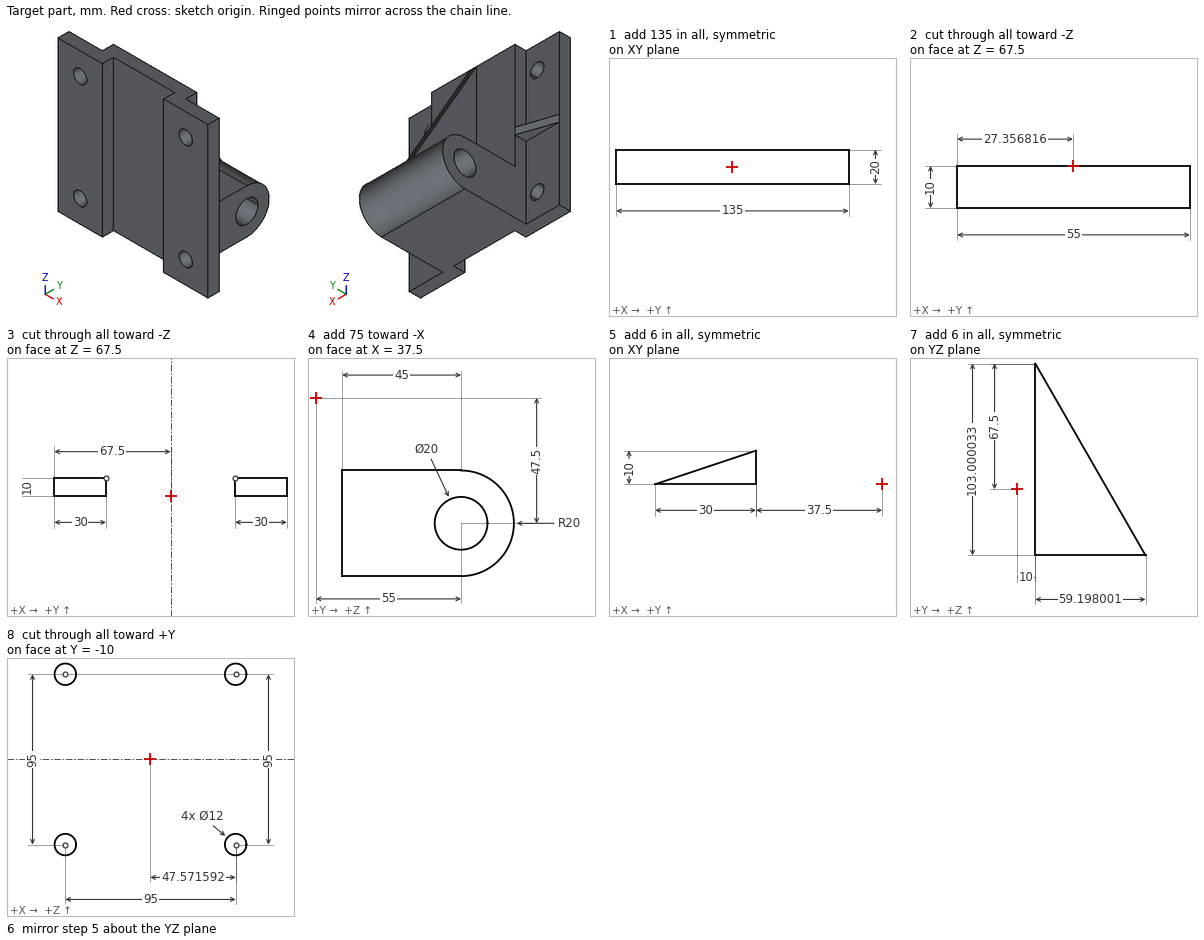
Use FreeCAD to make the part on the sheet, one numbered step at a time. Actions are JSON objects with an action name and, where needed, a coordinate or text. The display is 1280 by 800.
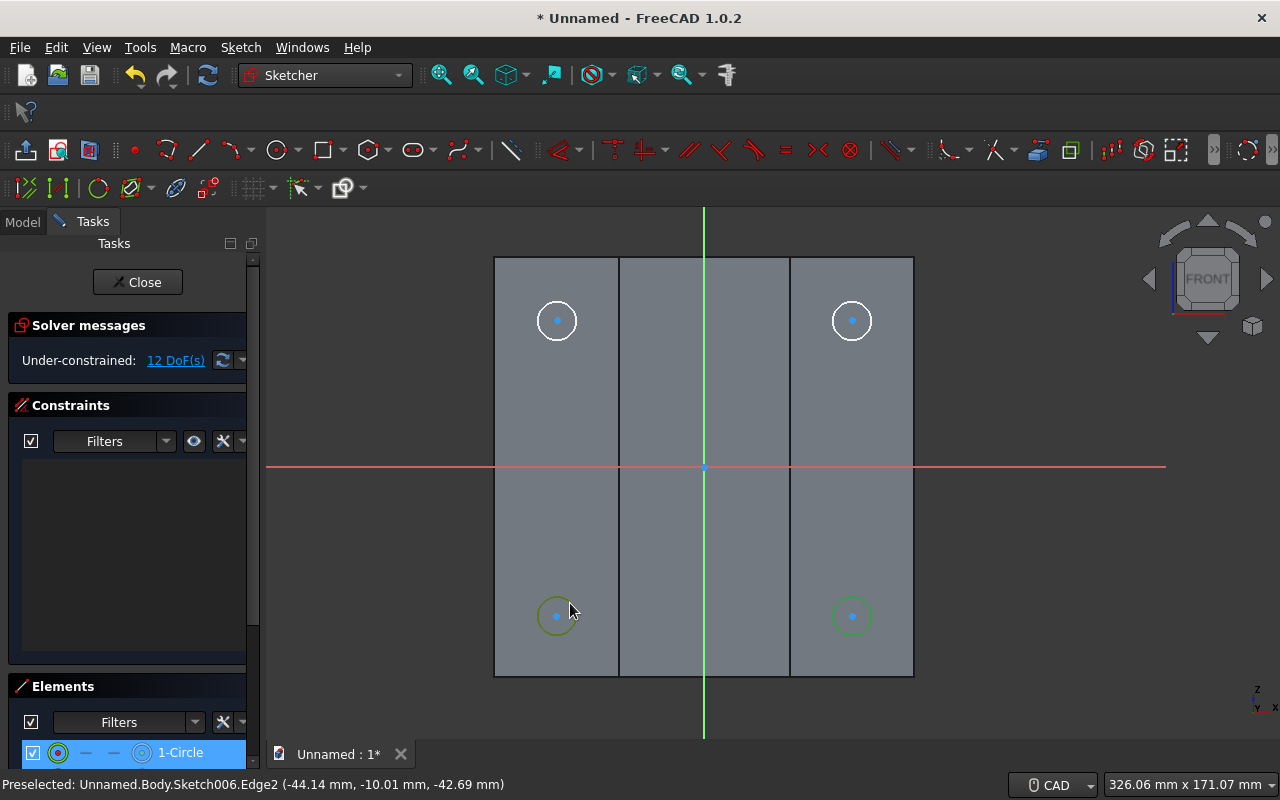
{"action": "left_click", "coordinate": [570, 307]}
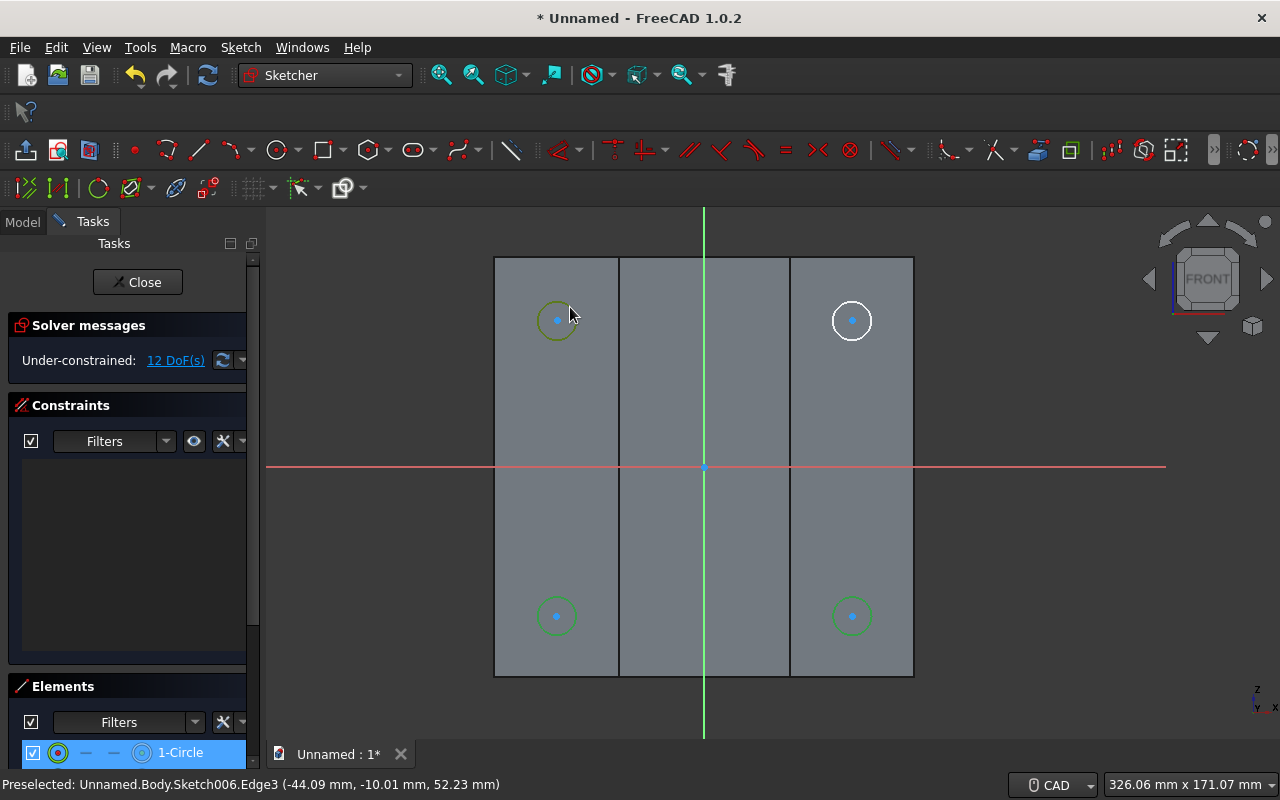
{"action": "left_click", "coordinate": [865, 307]}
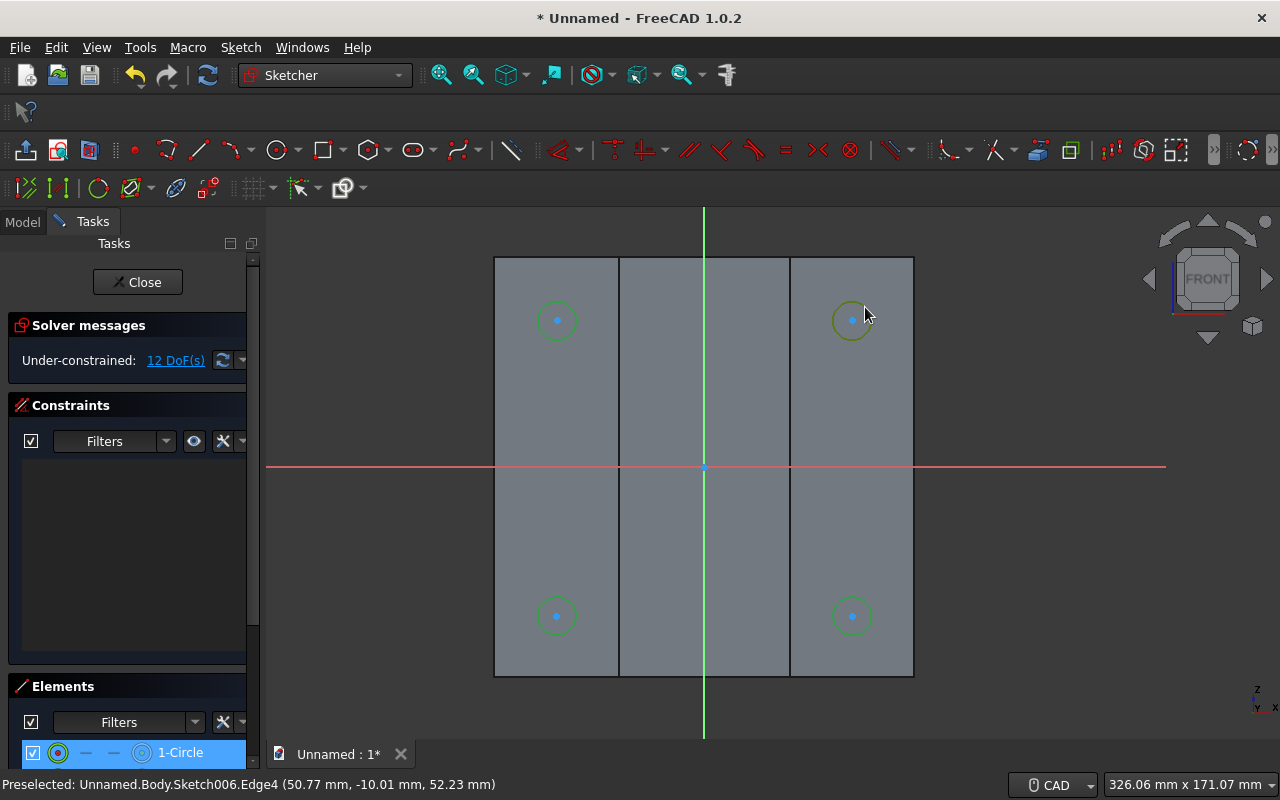
{"action": "left_click", "coordinate": [786, 150]}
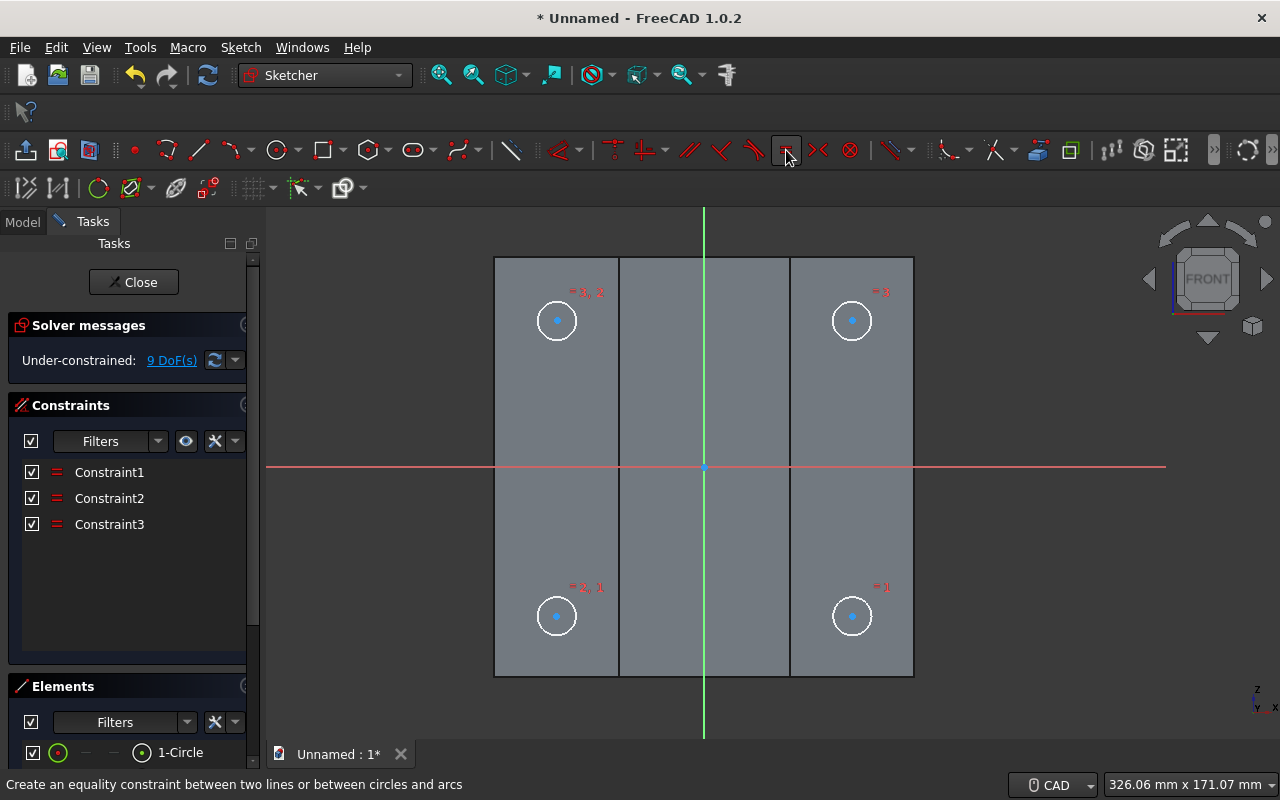
{"action": "left_click", "coordinate": [557, 616]}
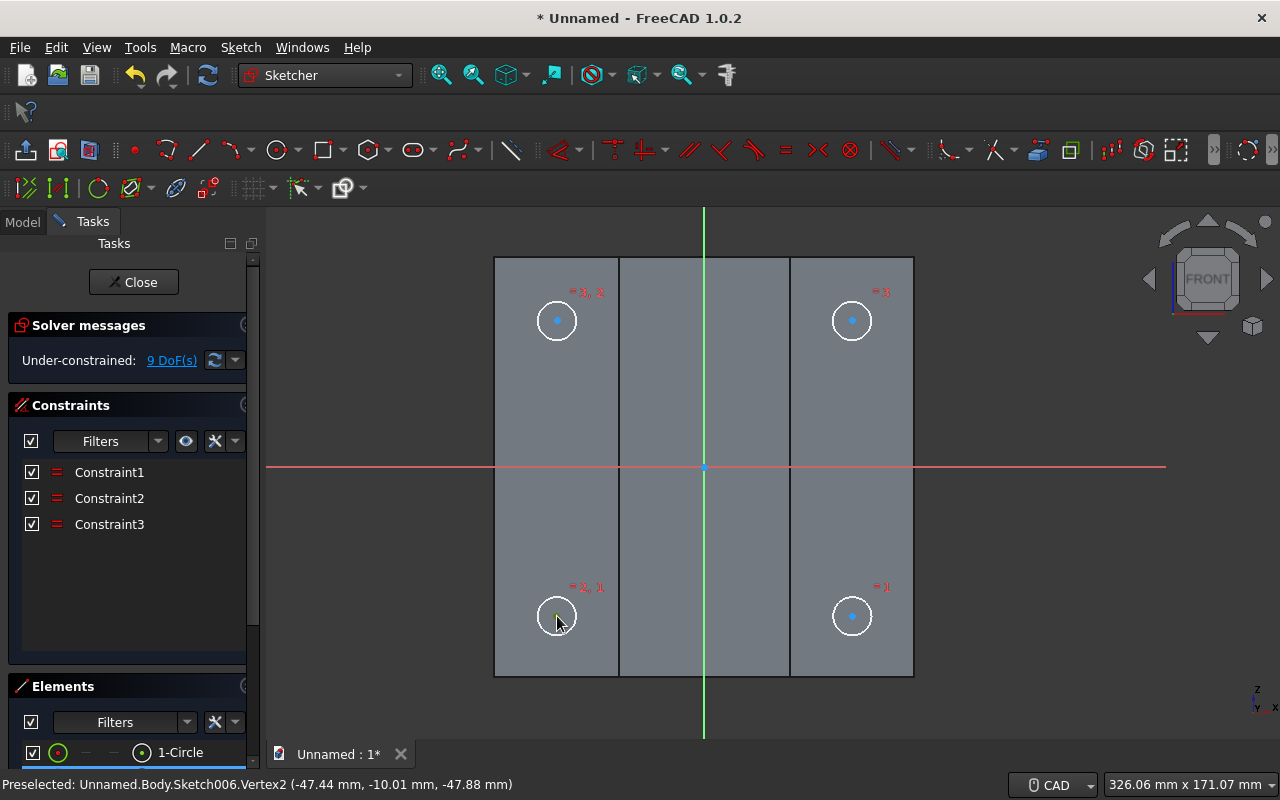
{"action": "left_click", "coordinate": [557, 321]}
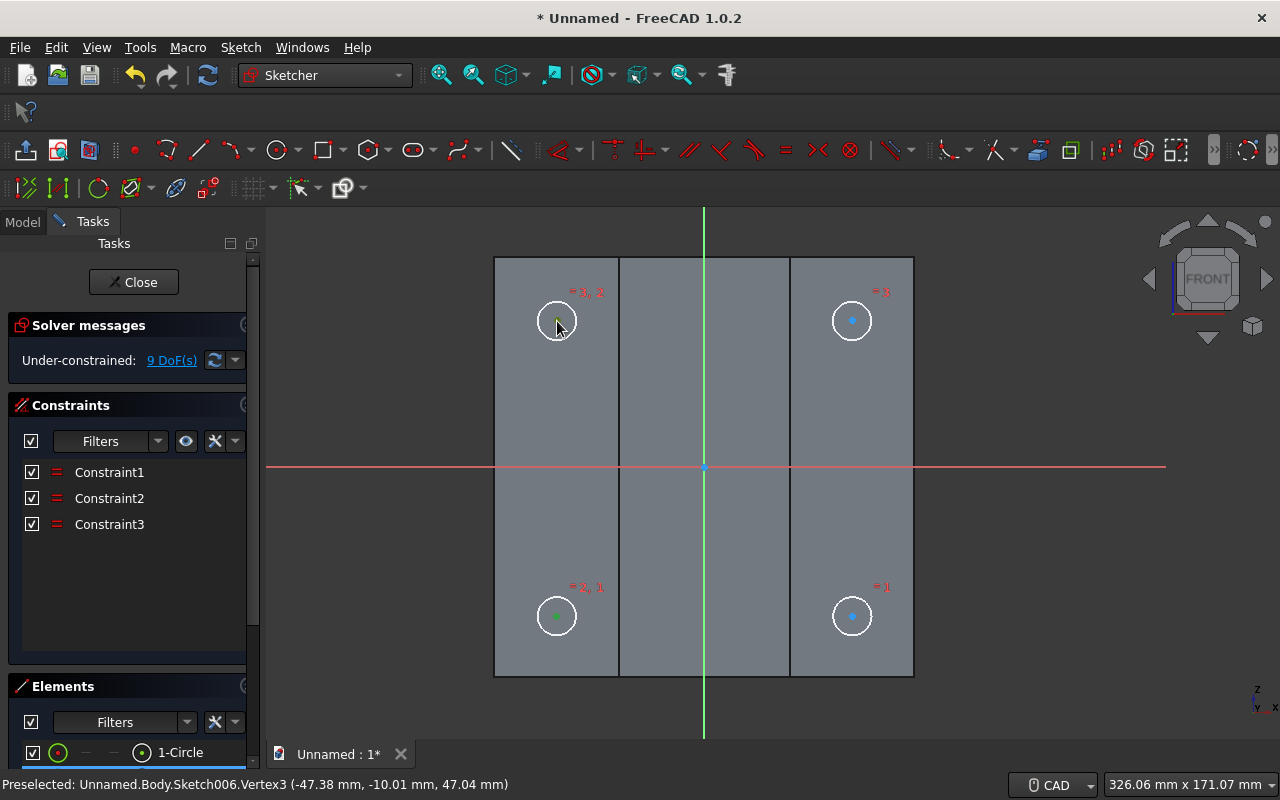
{"action": "left_click", "coordinate": [353, 467]}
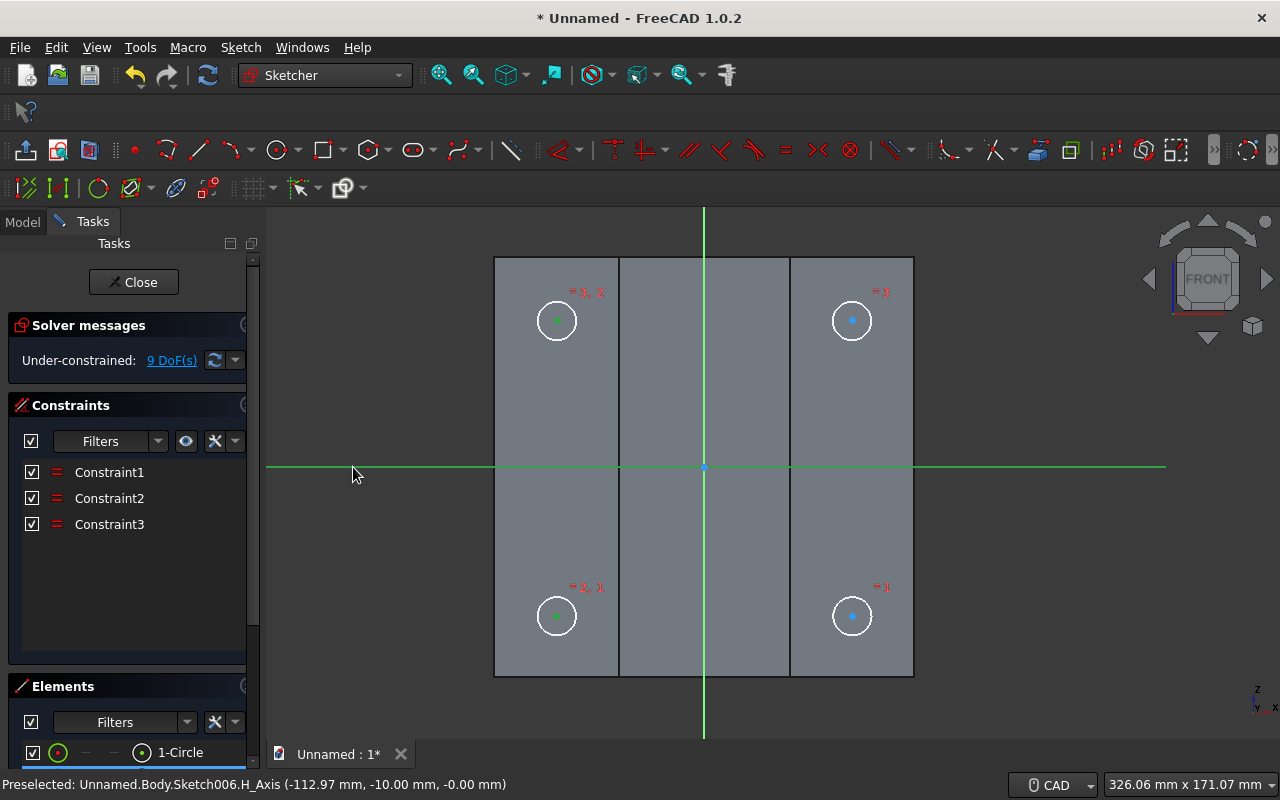
{"action": "left_click", "coordinate": [818, 150]}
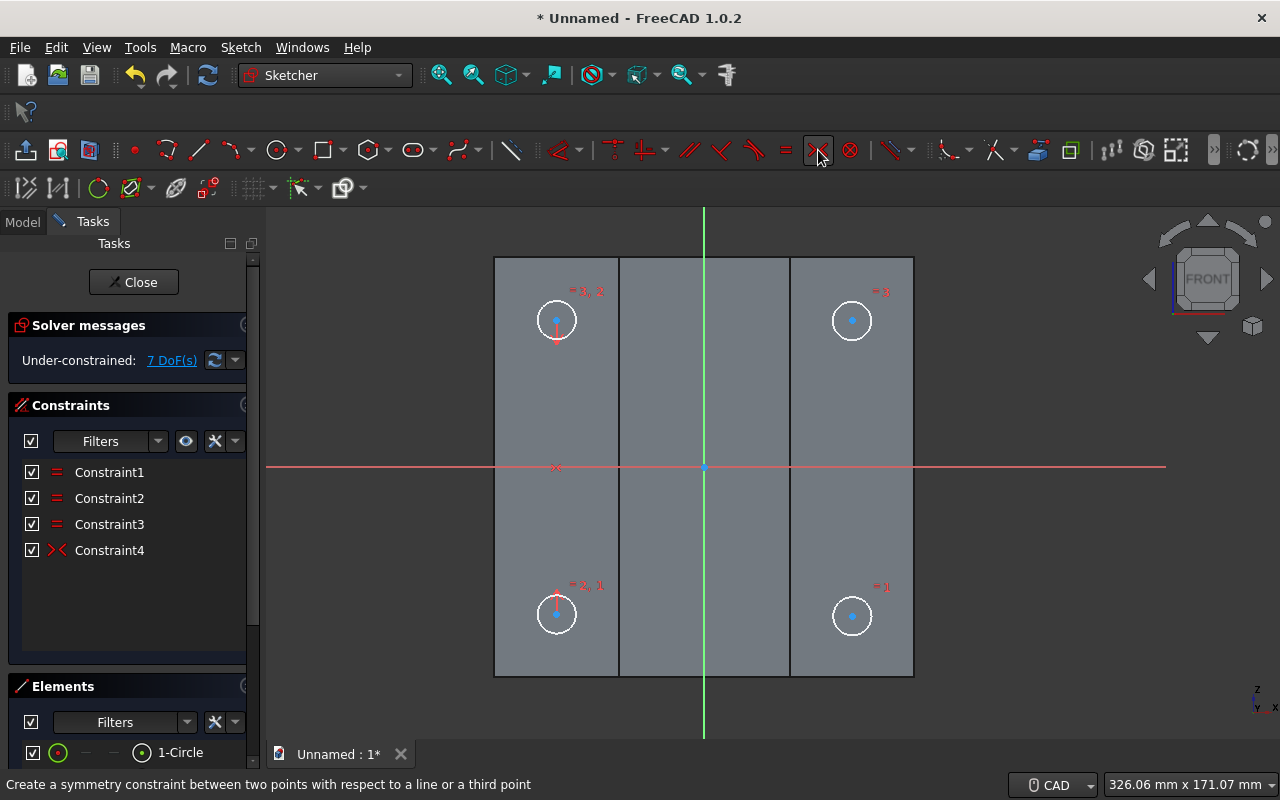
{"action": "left_click", "coordinate": [852, 616]}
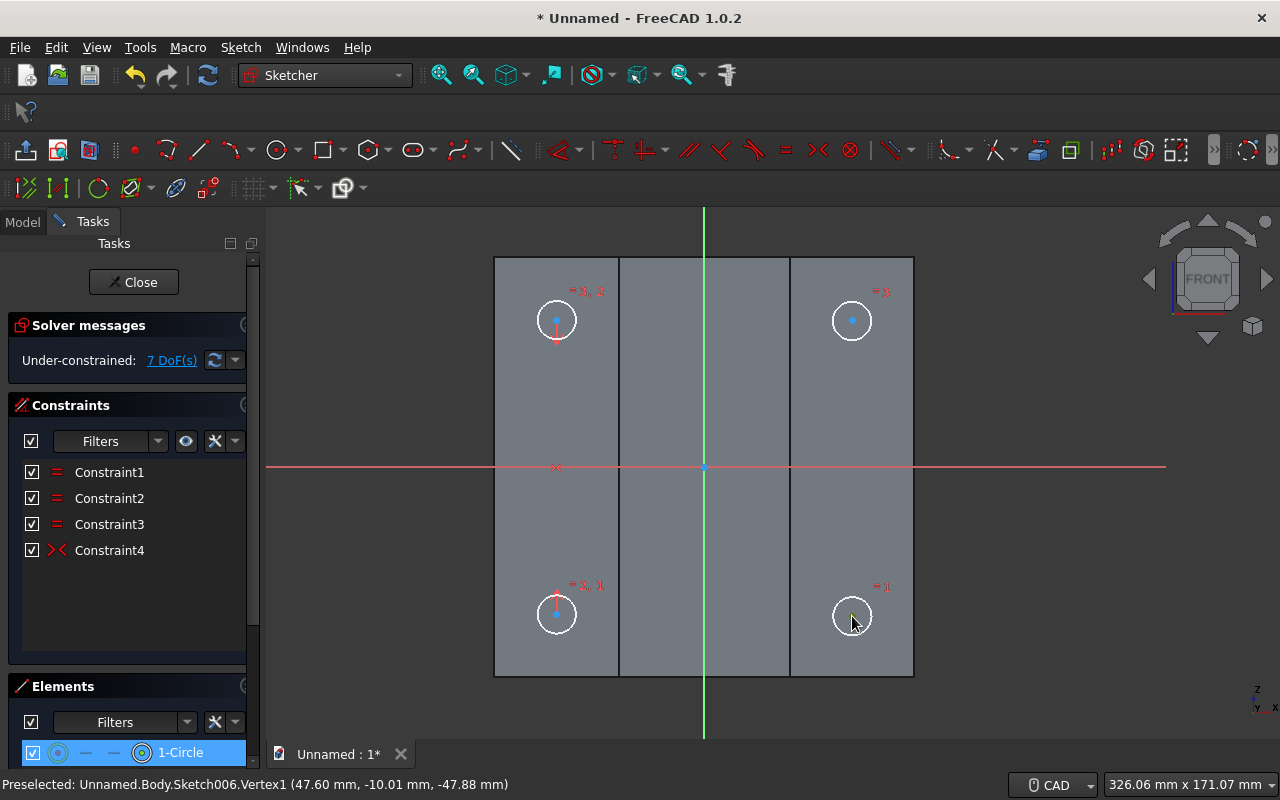
{"action": "left_click", "coordinate": [852, 321]}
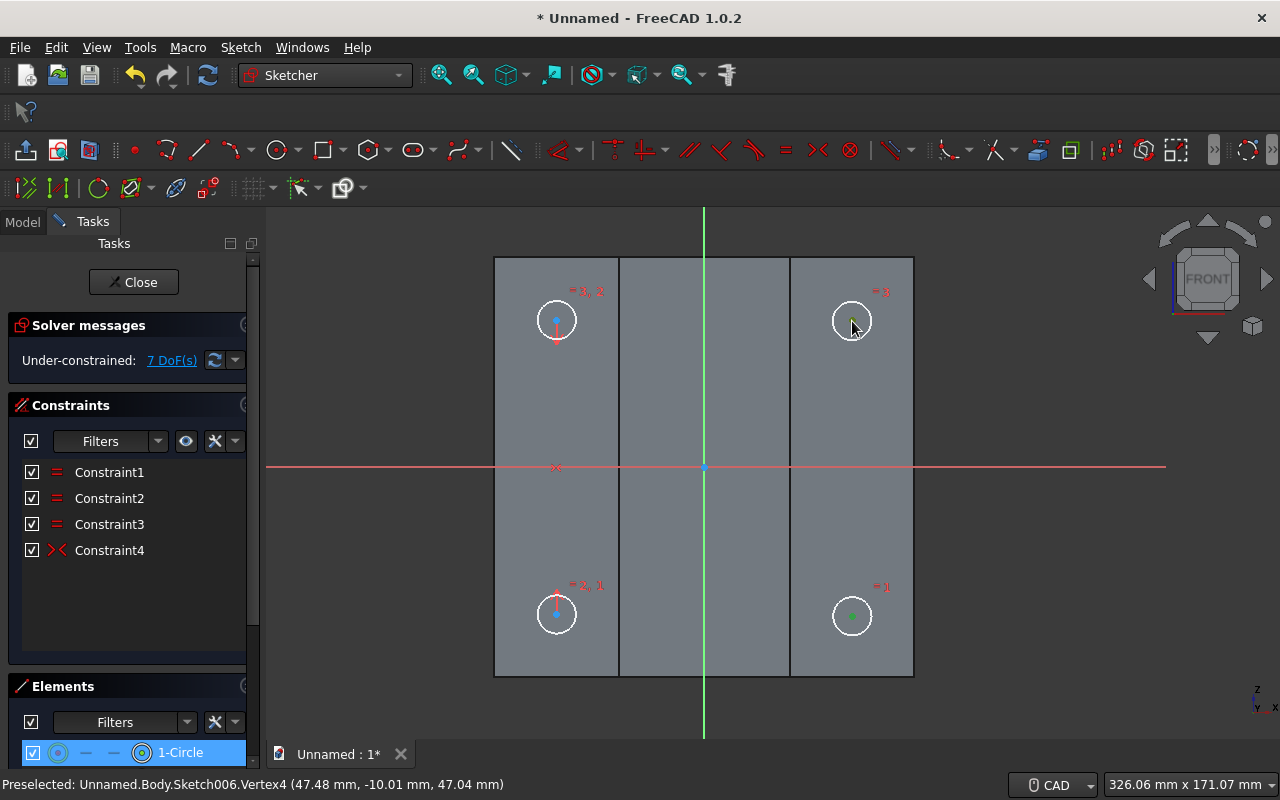
{"action": "left_click", "coordinate": [353, 467]}